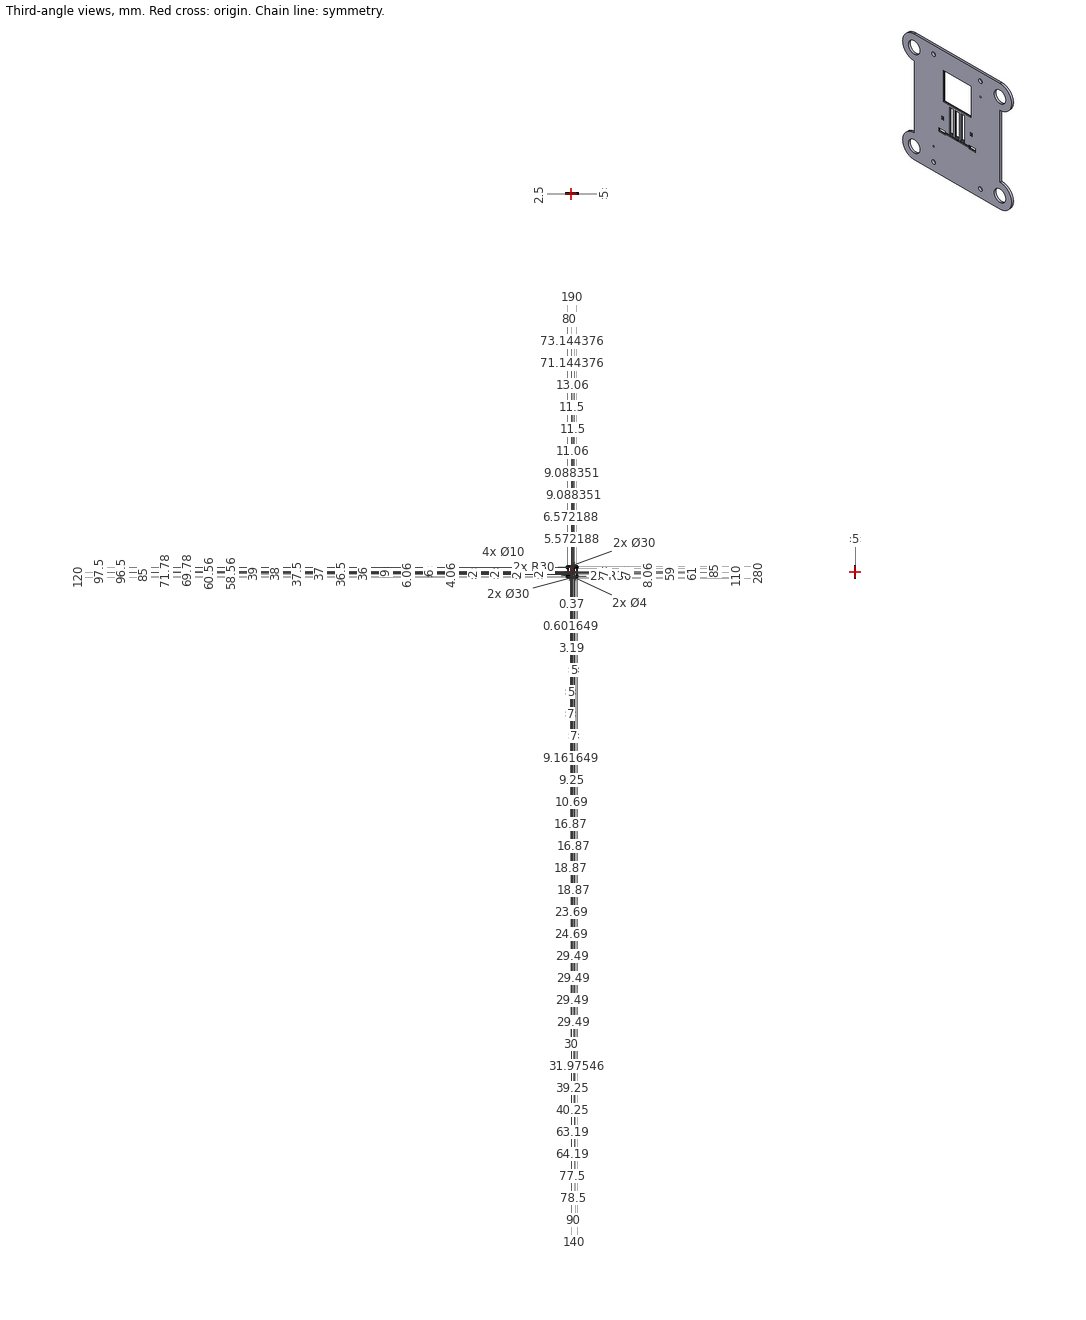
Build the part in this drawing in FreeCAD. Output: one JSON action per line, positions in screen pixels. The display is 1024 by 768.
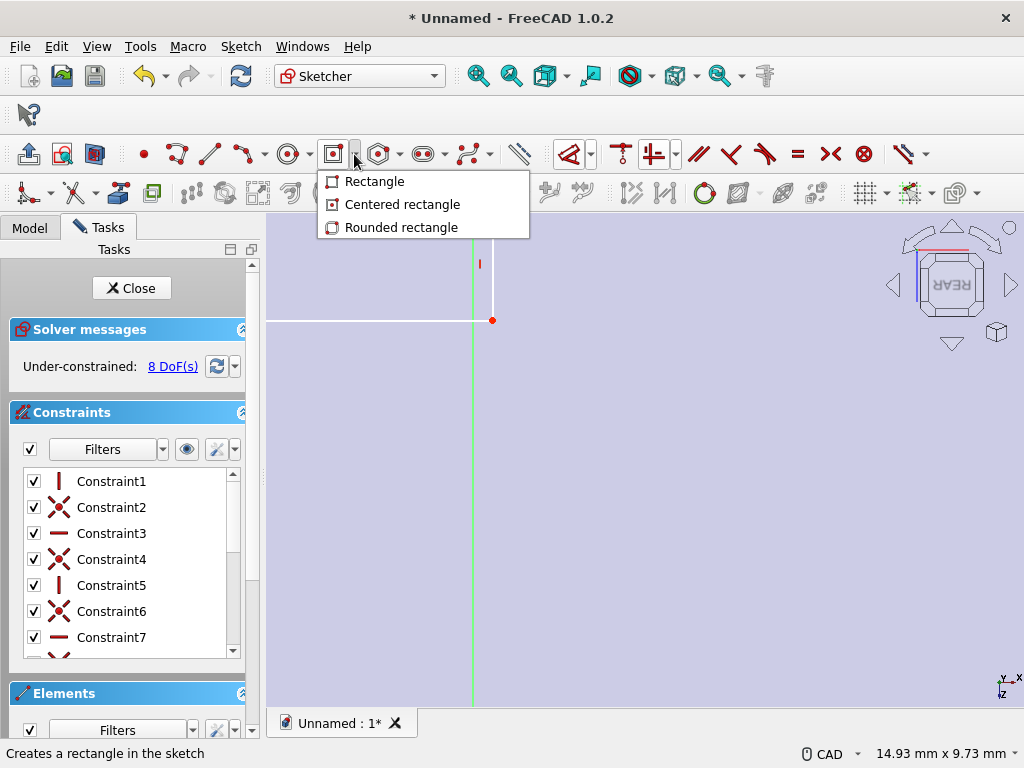
{"action": "left_click", "coordinate": [424, 182]}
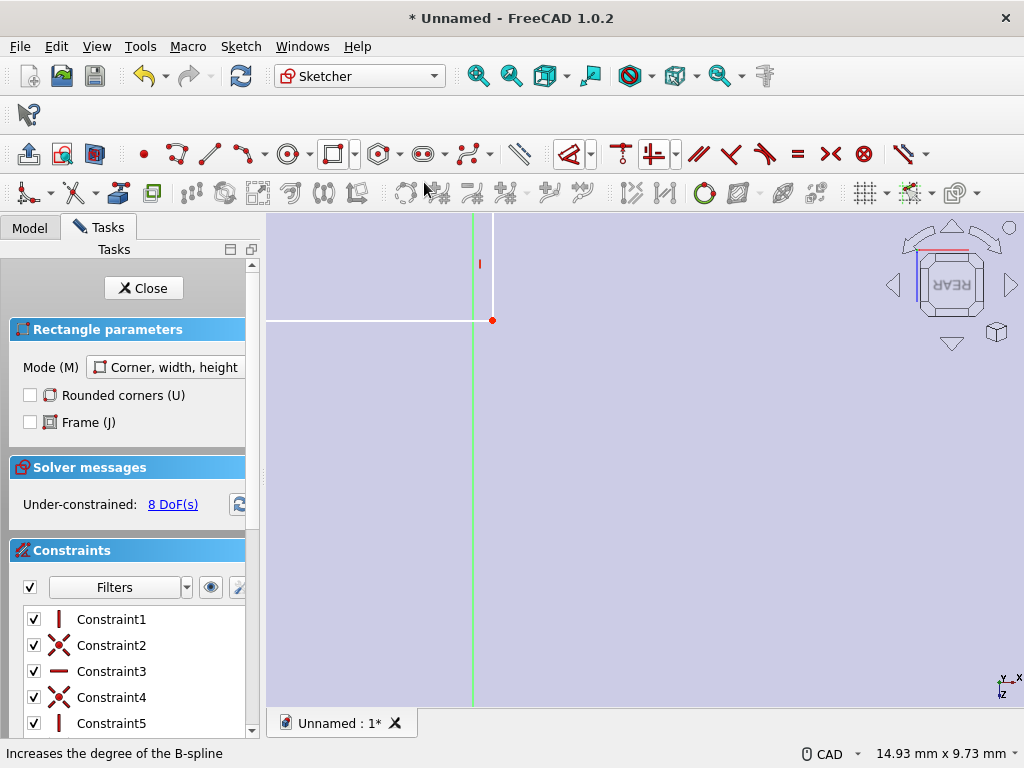
{"action": "scroll", "coordinate": [502, 304], "scroll_direction": "down", "scroll_amount": 15}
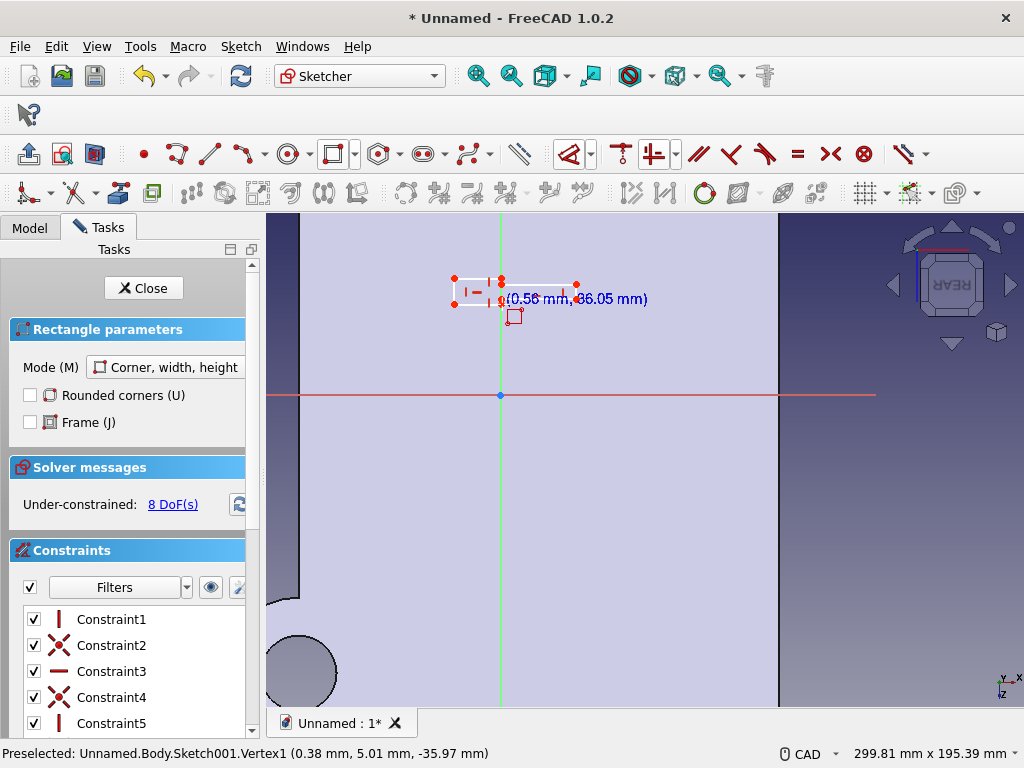
{"action": "left_click", "coordinate": [484, 460]}
{"action": "left_click", "coordinate": [669, 642]}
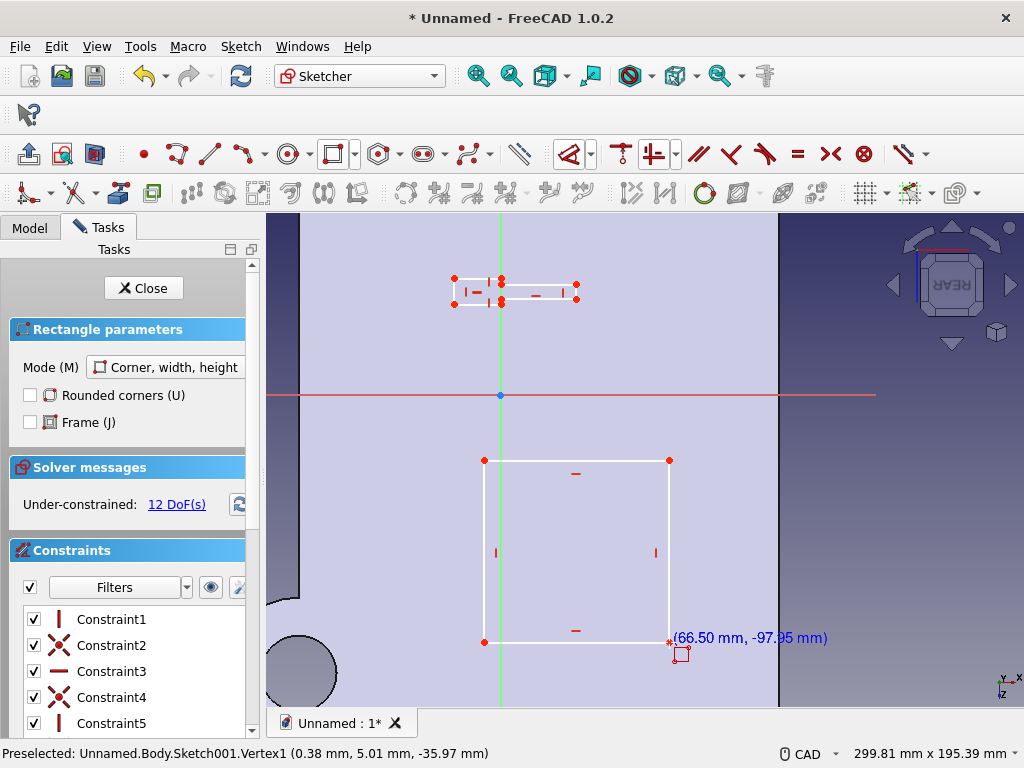
{"action": "left_click", "coordinate": [475, 357]}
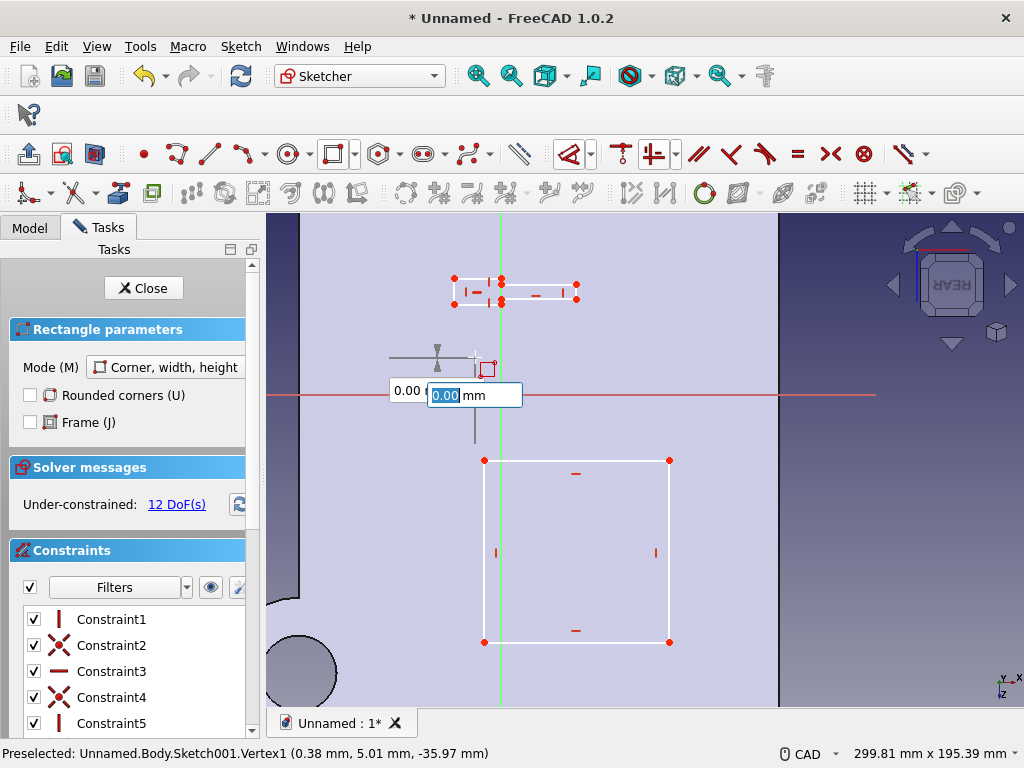
{"action": "scroll", "coordinate": [493, 380], "scroll_direction": "up", "scroll_amount": 4}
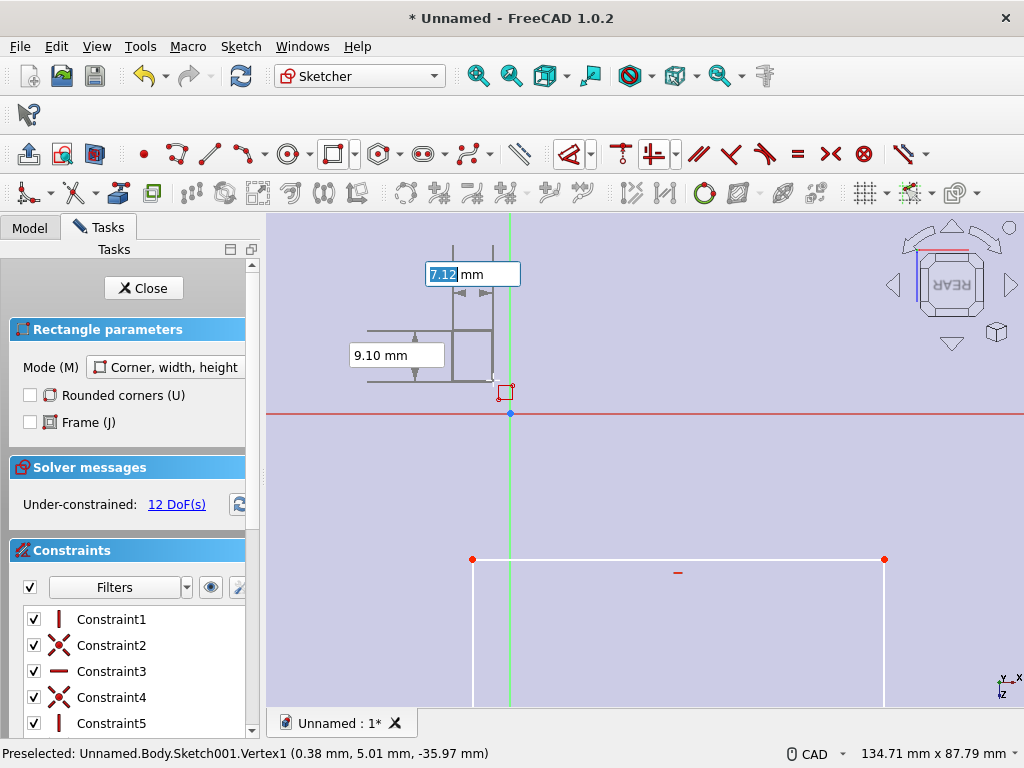
{"action": "left_click", "coordinate": [492, 380]}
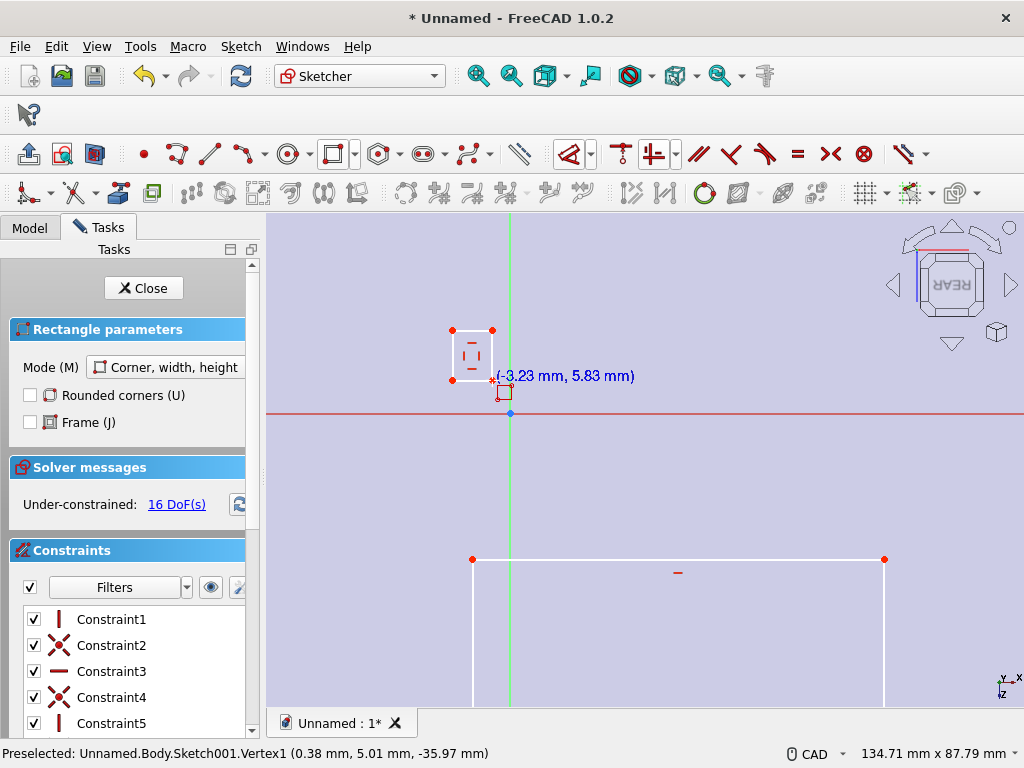
{"action": "scroll", "coordinate": [517, 403], "scroll_direction": "down", "scroll_amount": 5}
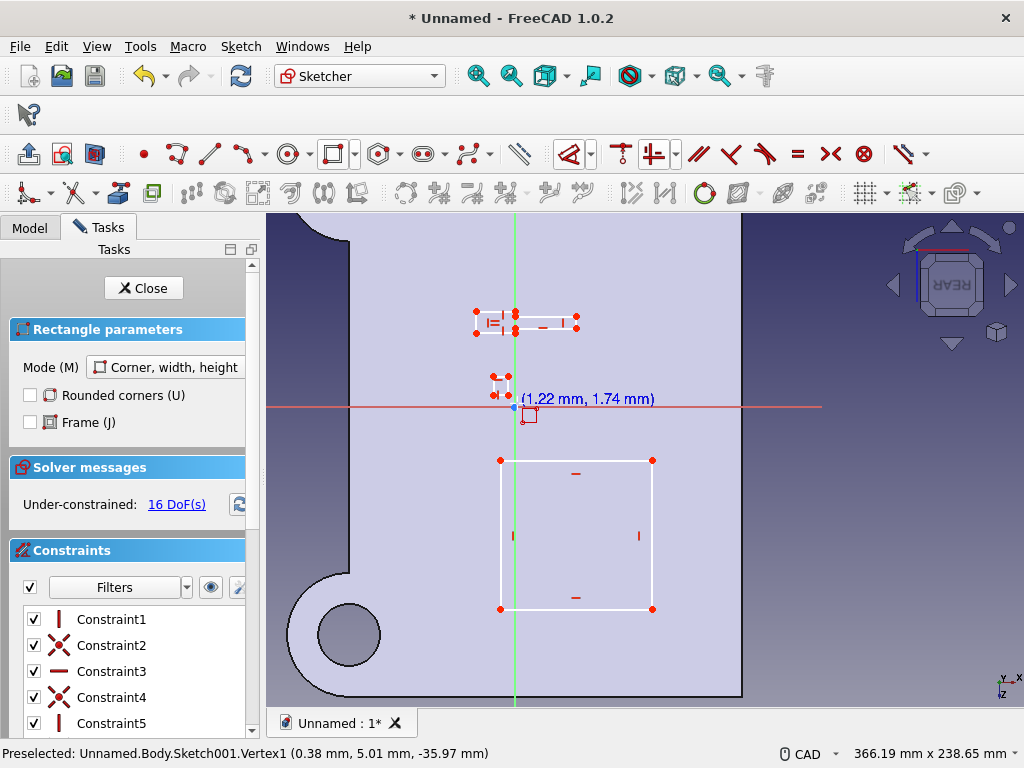
{"action": "left_click", "coordinate": [645, 376]}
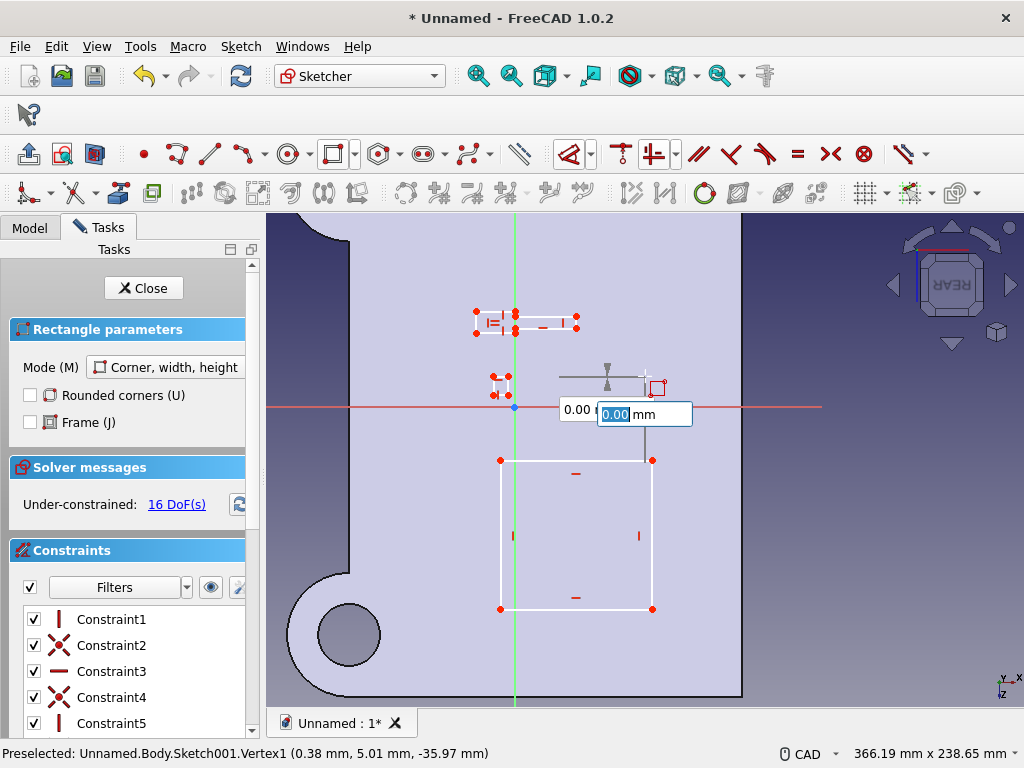
{"action": "scroll", "coordinate": [660, 395], "scroll_direction": "up", "scroll_amount": 2}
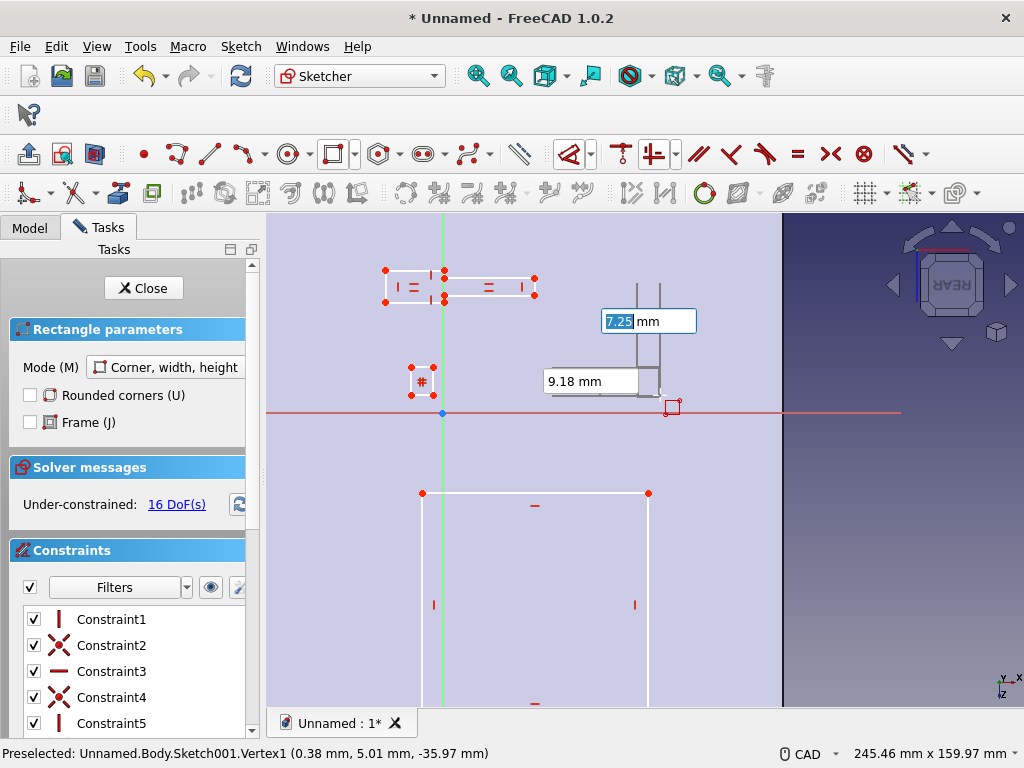
{"action": "left_click", "coordinate": [660, 395]}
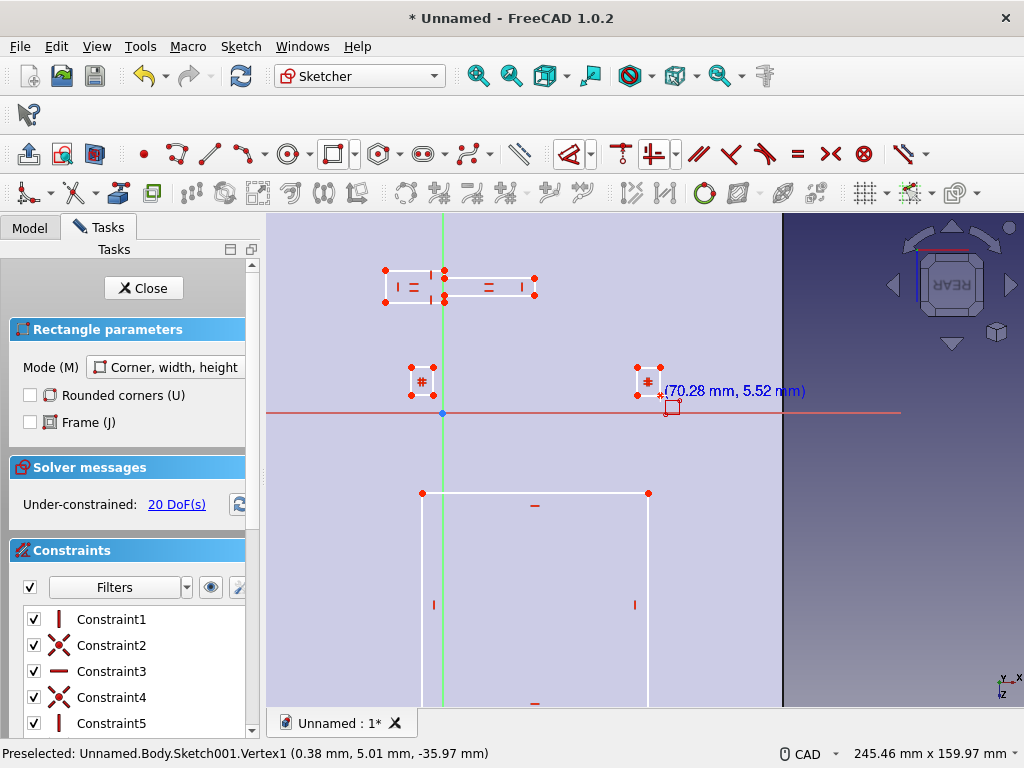
{"action": "left_click", "coordinate": [564, 297]}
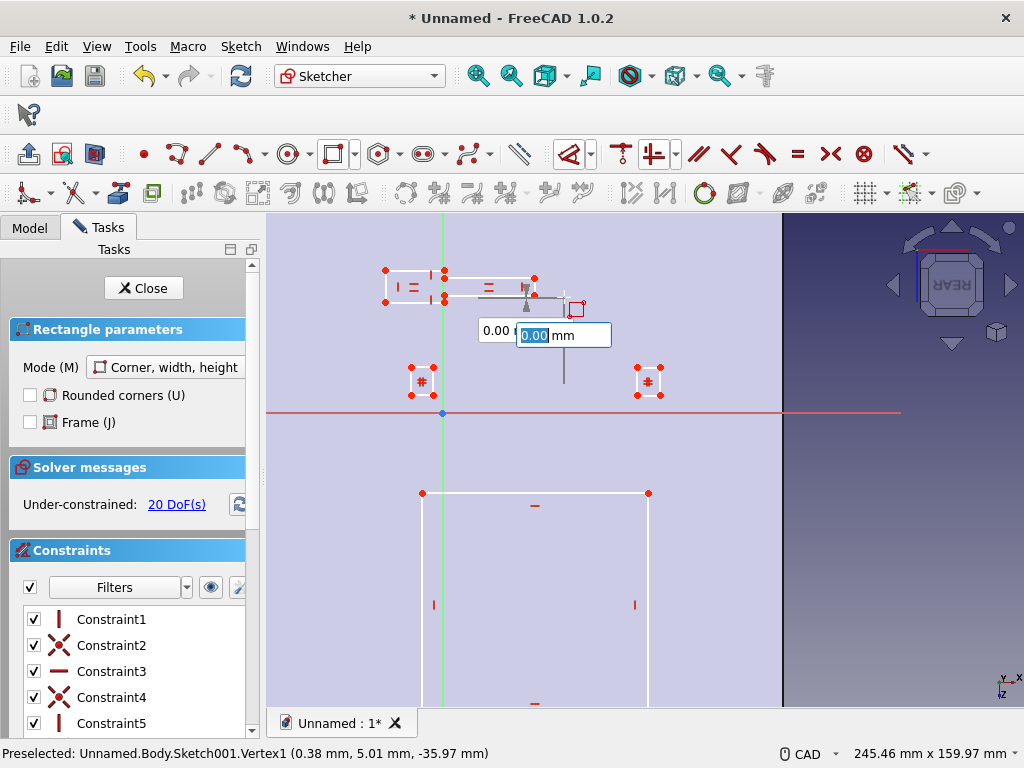
{"action": "scroll", "coordinate": [600, 486], "scroll_direction": "up", "scroll_amount": 5}